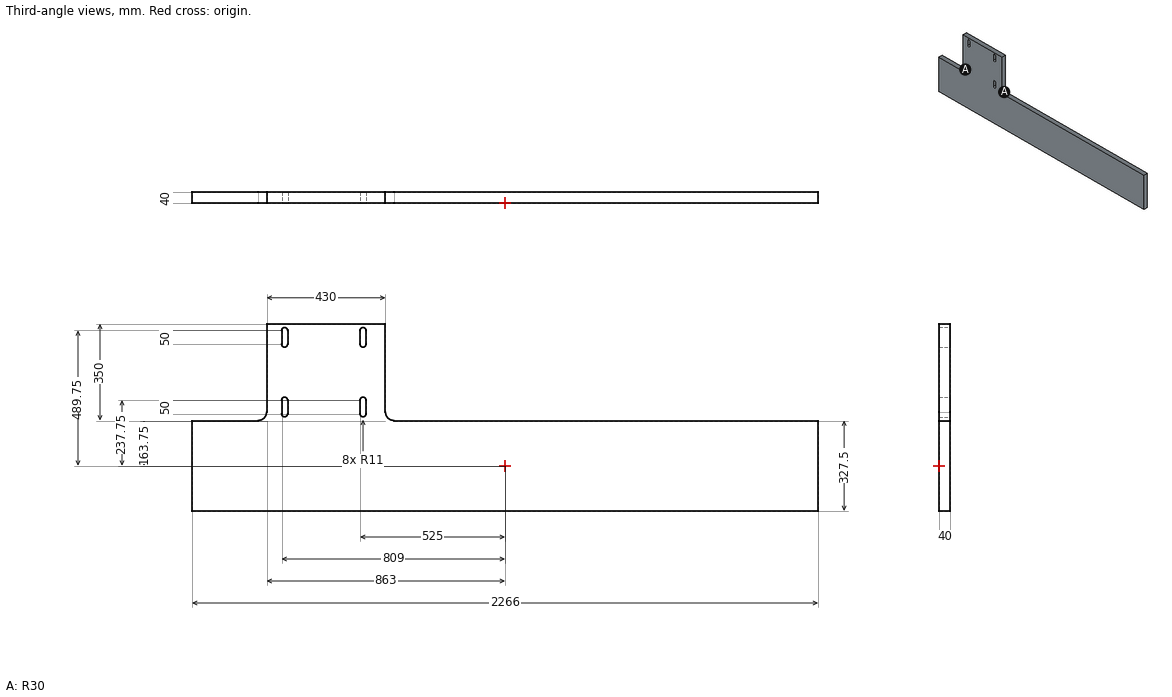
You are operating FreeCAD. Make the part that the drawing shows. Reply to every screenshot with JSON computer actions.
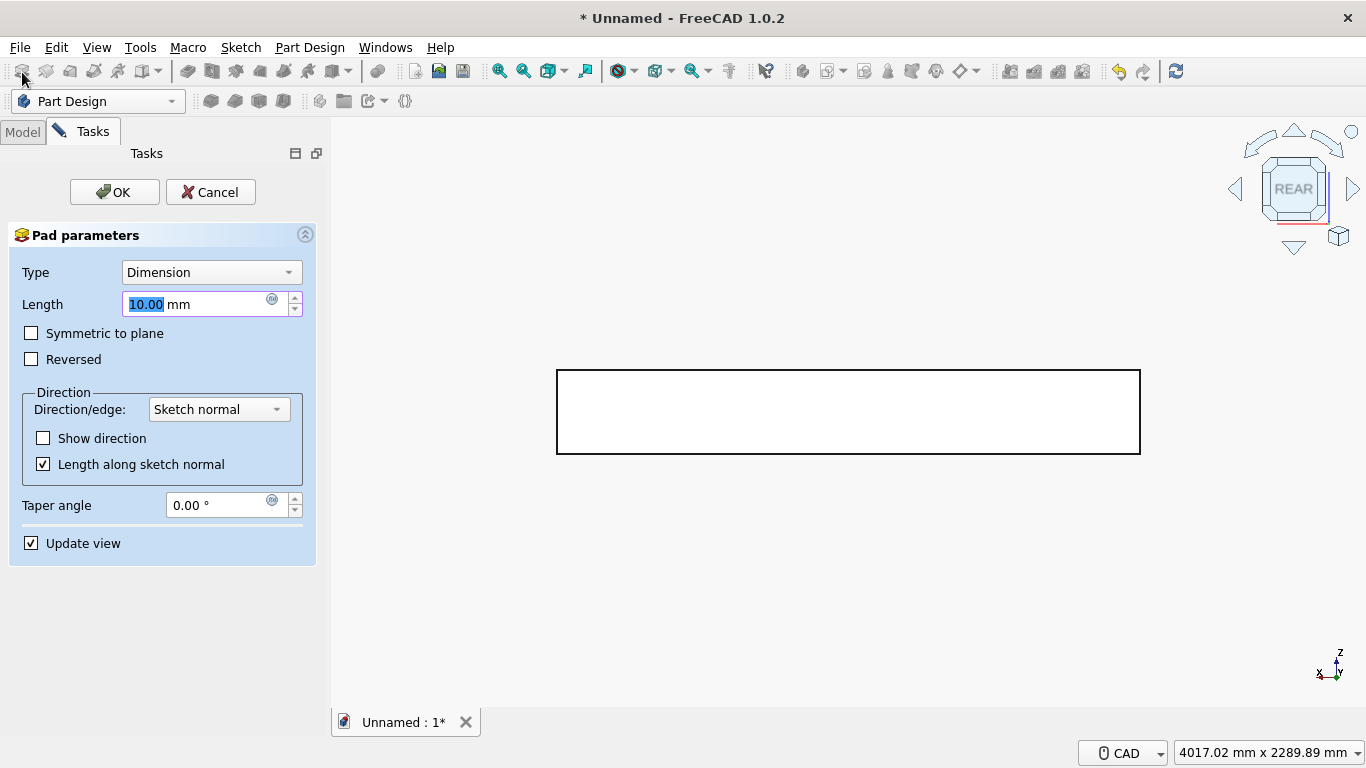
{"action": "type", "text": "40"}
{"action": "key", "text": "Tab"}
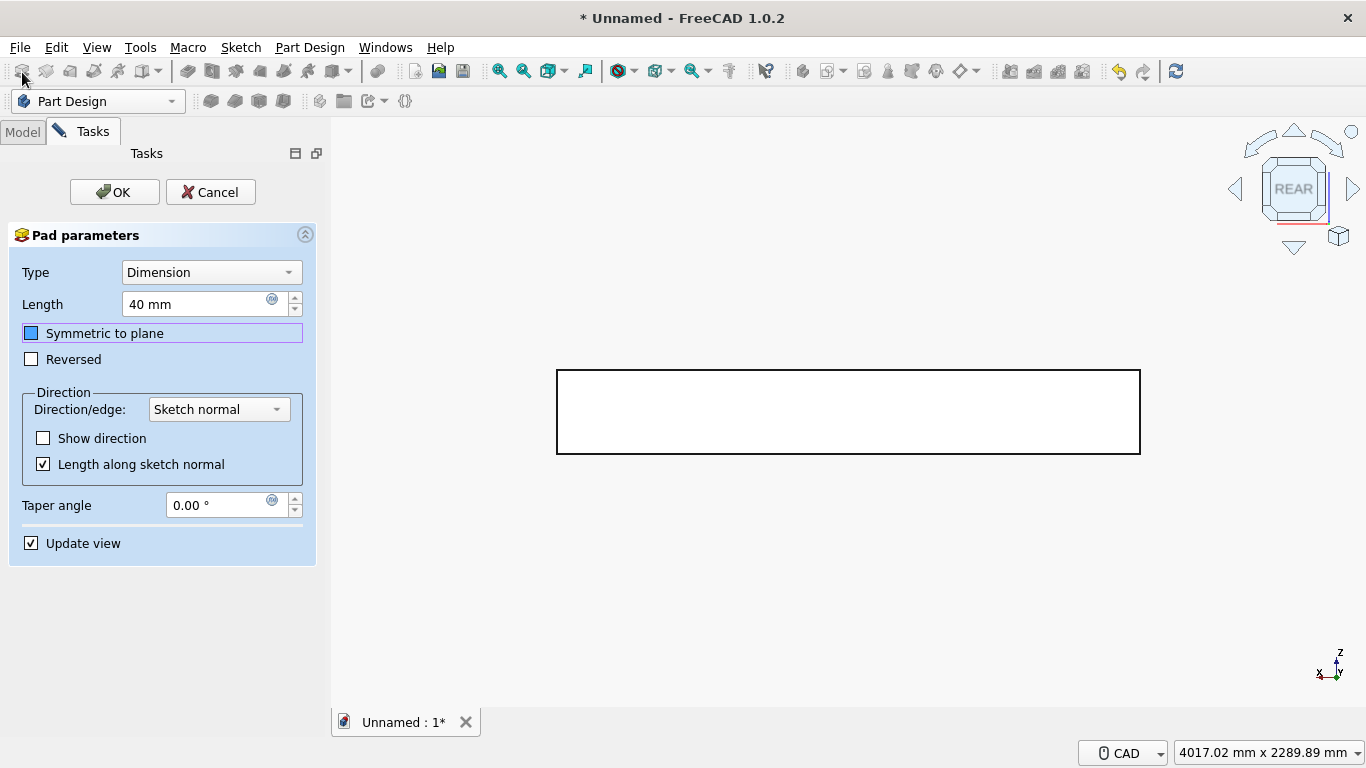
{"action": "left_click", "coordinate": [30, 359]}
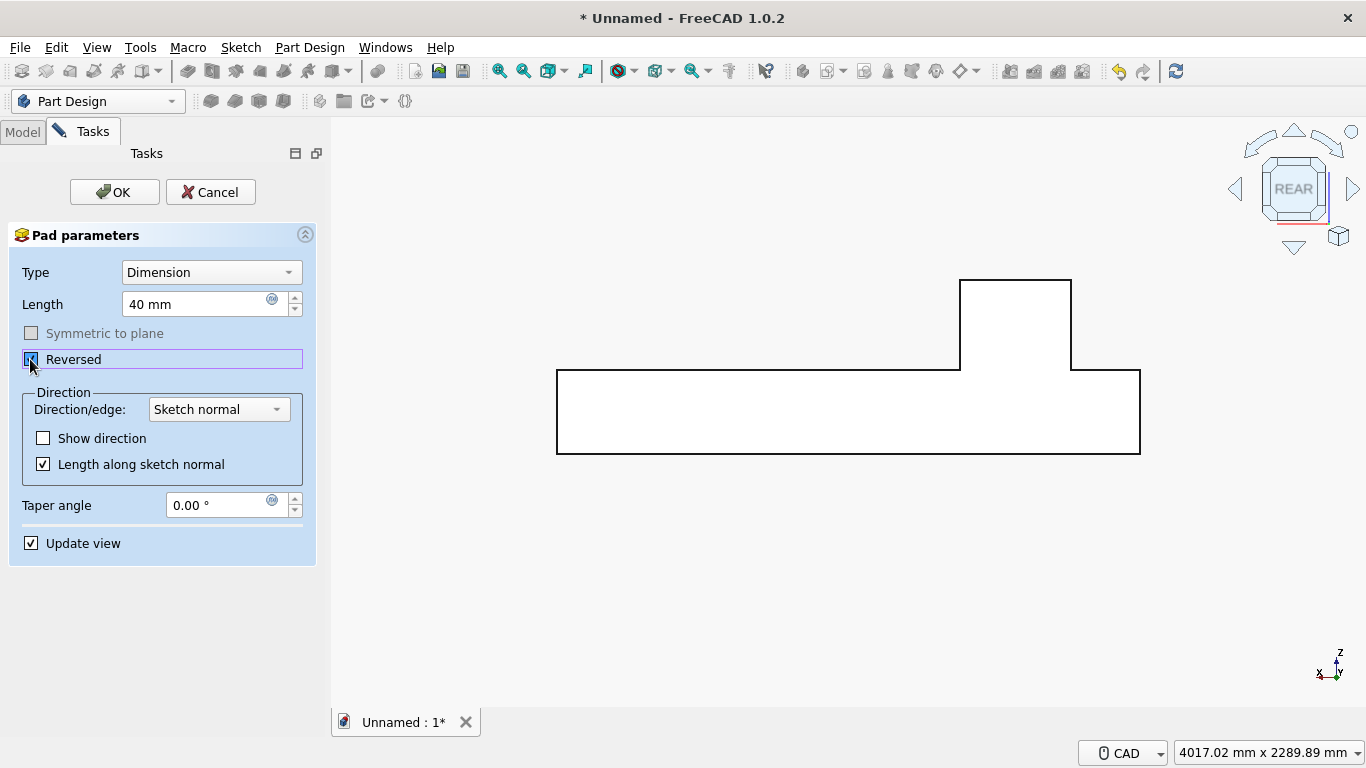
{"action": "left_click", "coordinate": [115, 192]}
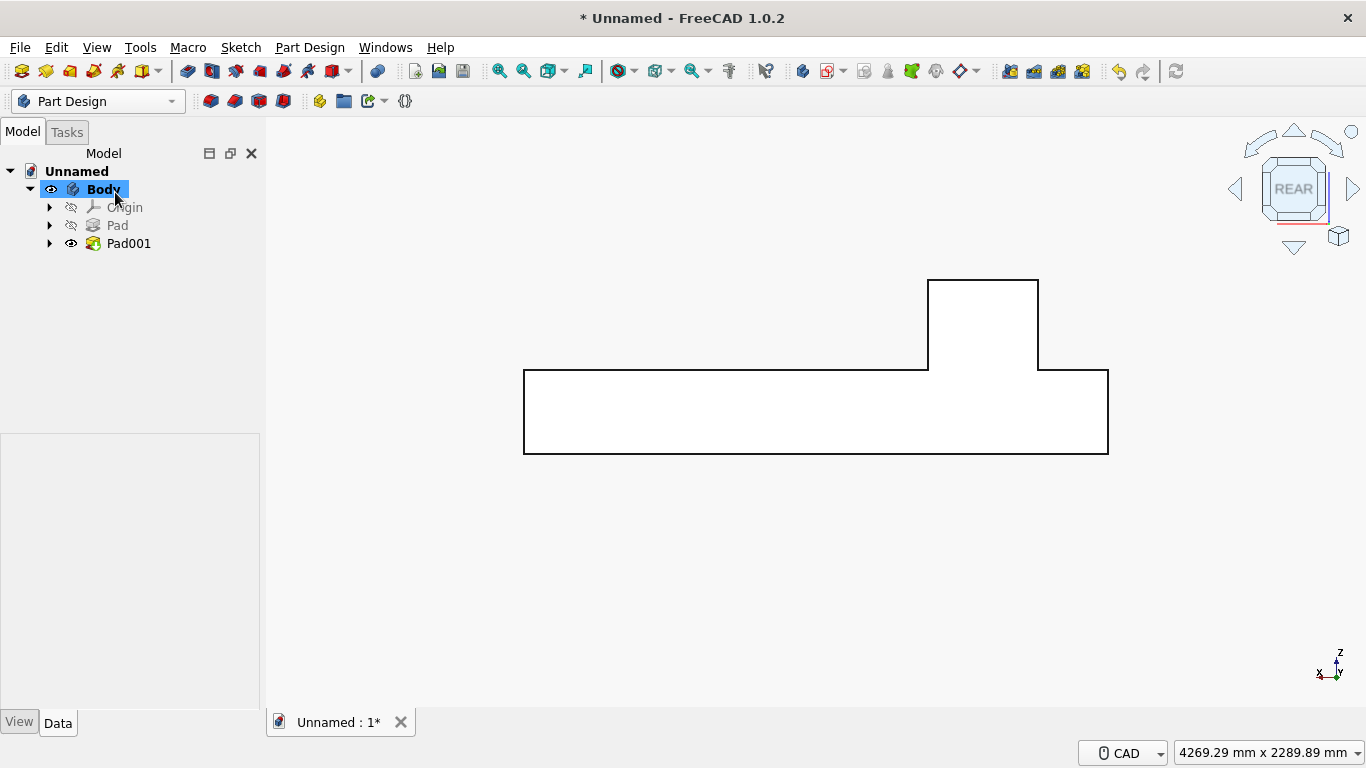
{"action": "left_click", "coordinate": [983, 391]}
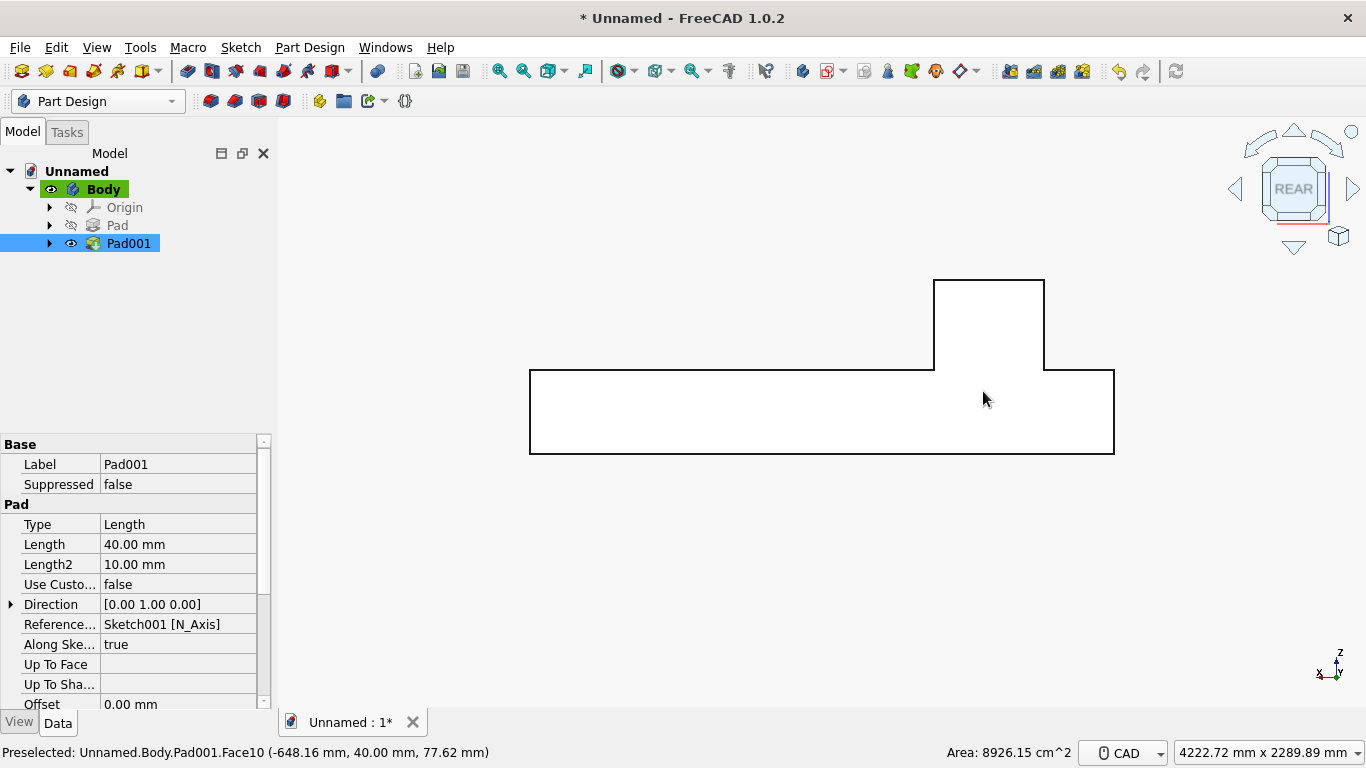
{"action": "left_click", "coordinate": [828, 72]}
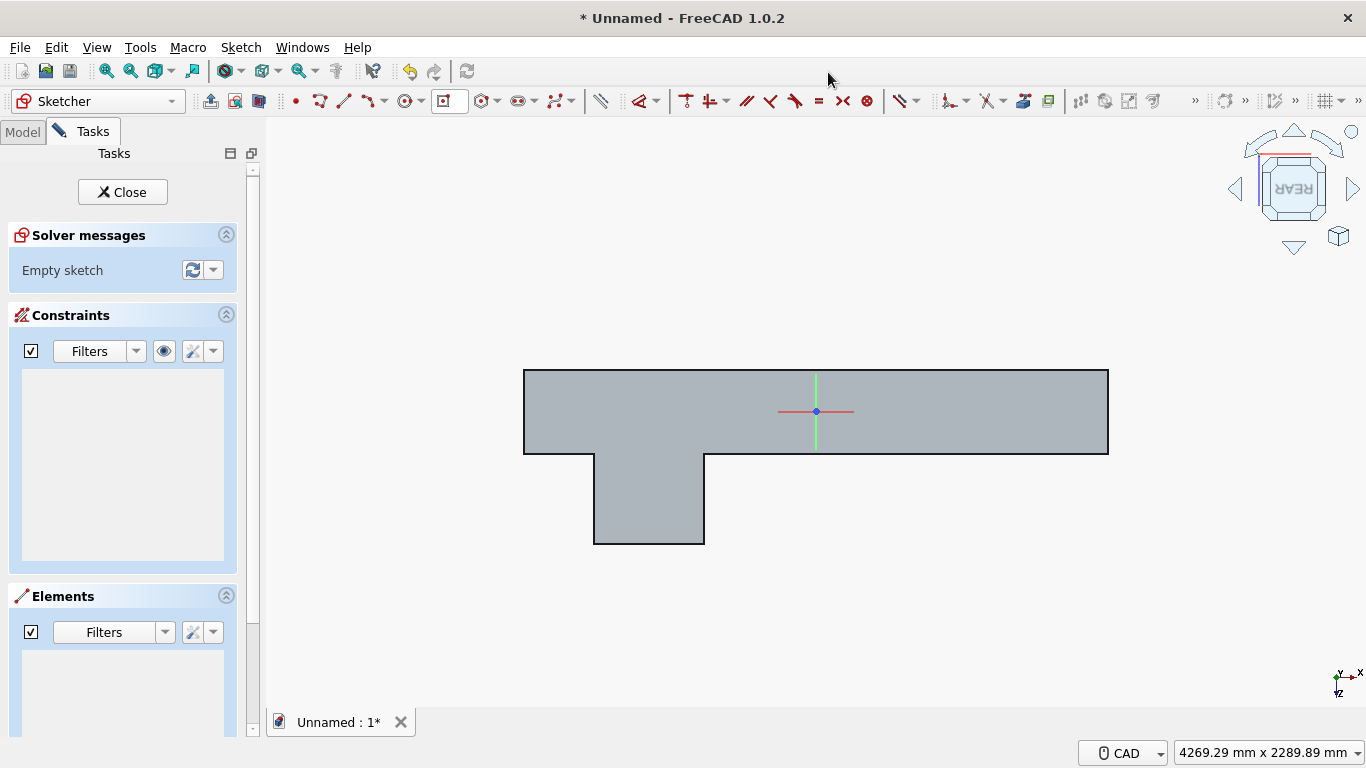
{"action": "scroll", "coordinate": [691, 514], "scroll_direction": "up", "scroll_amount": 5}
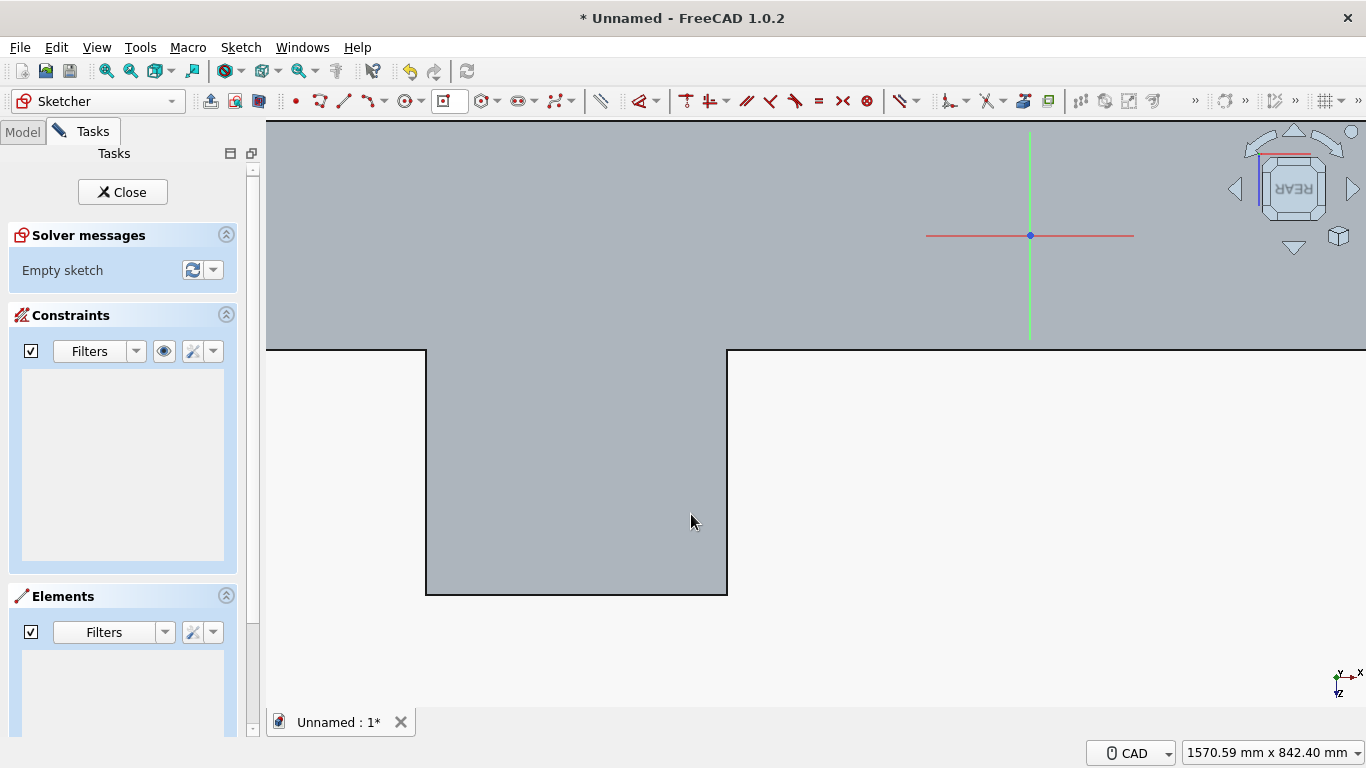
{"action": "left_click", "coordinate": [518, 102]}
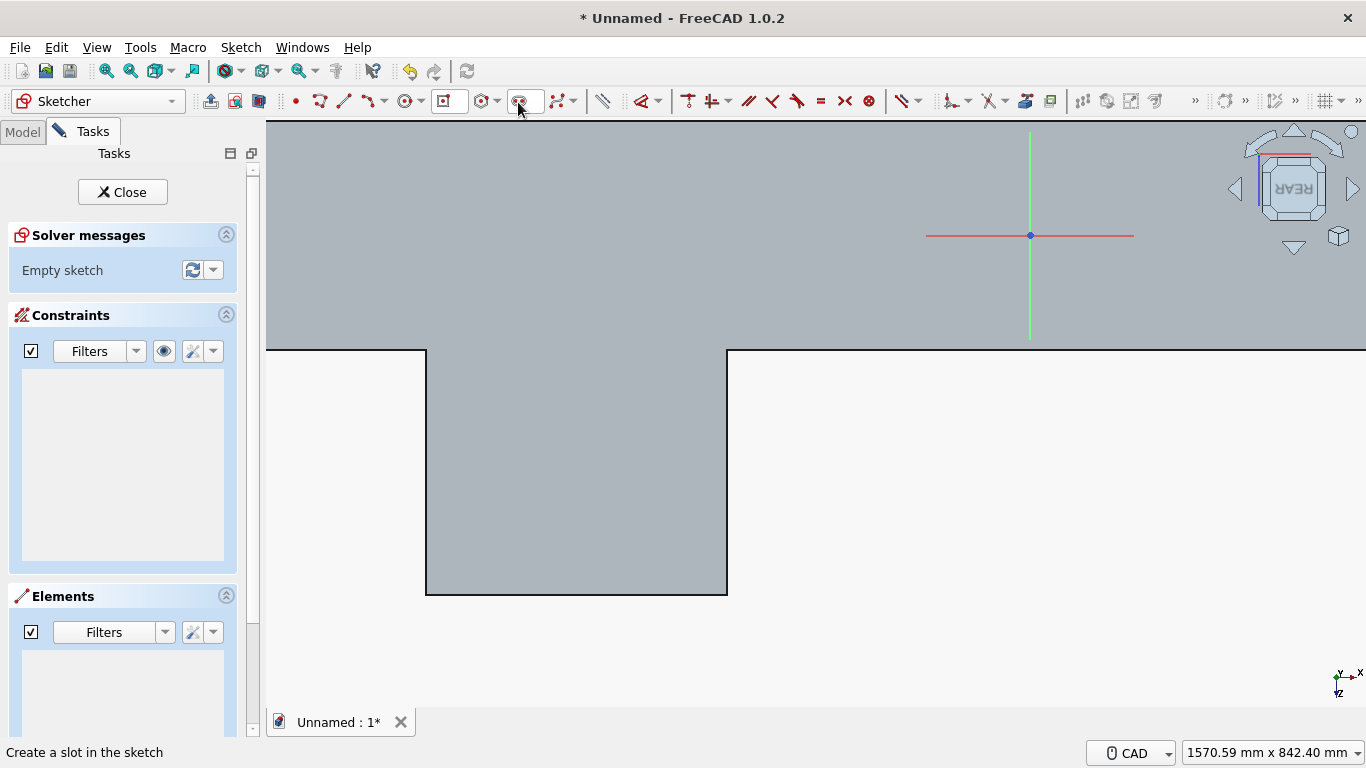
{"action": "scroll", "coordinate": [670, 402], "scroll_direction": "up", "scroll_amount": 6}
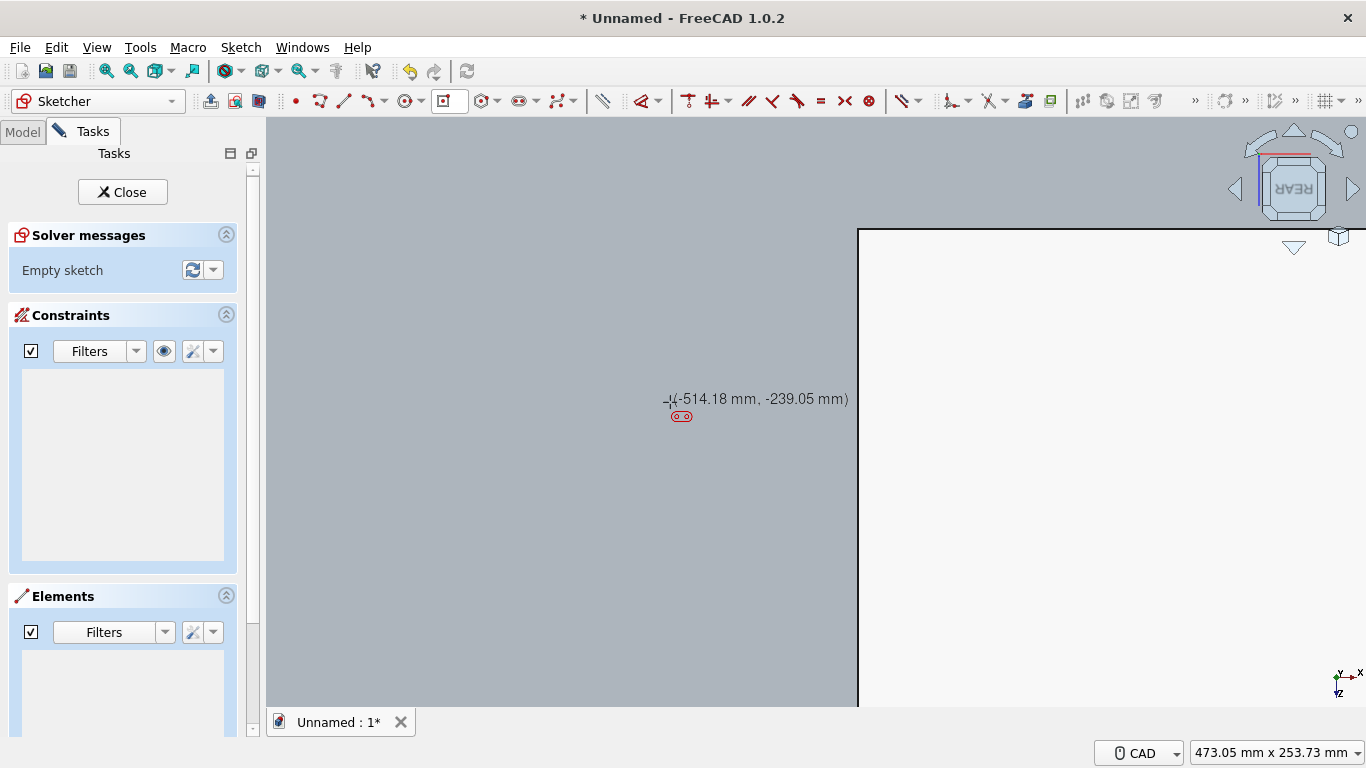
{"action": "left_click", "coordinate": [670, 401]}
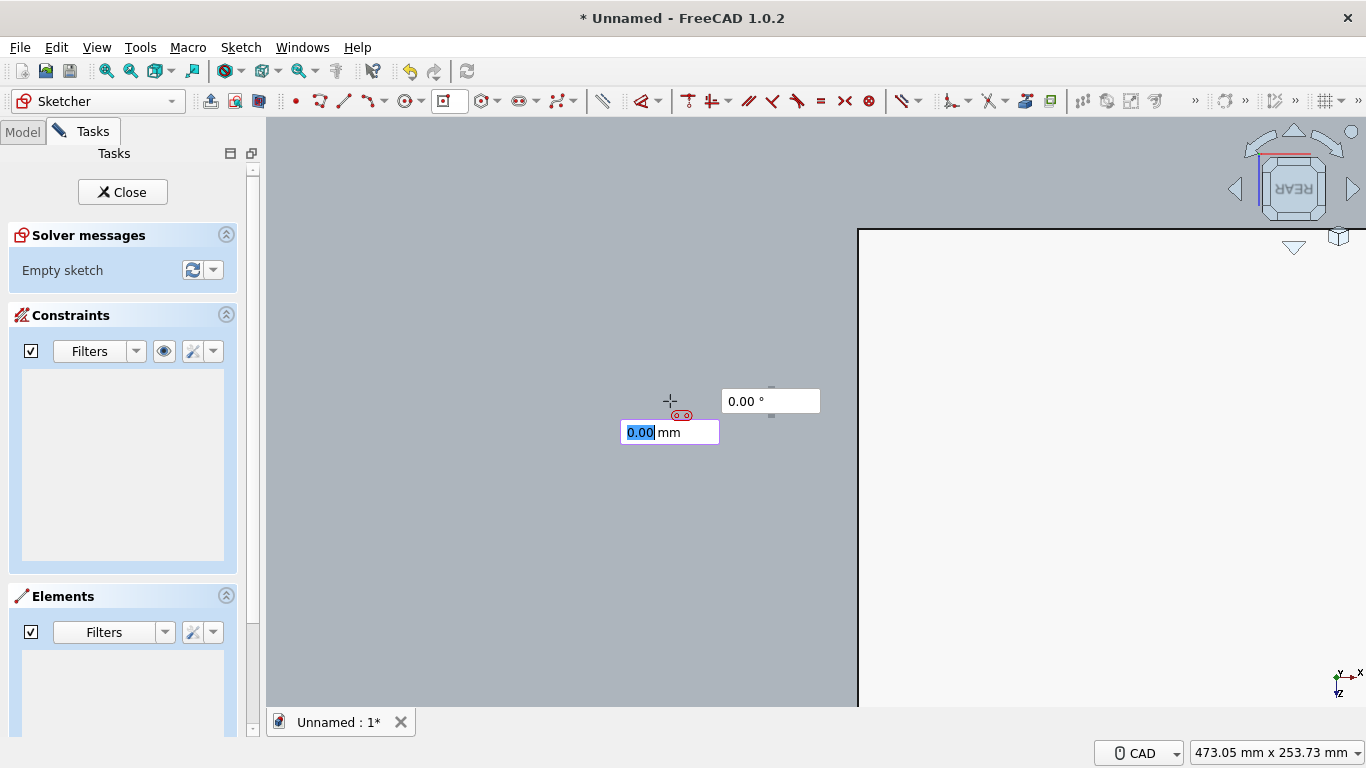
{"action": "left_click", "coordinate": [670, 285]}